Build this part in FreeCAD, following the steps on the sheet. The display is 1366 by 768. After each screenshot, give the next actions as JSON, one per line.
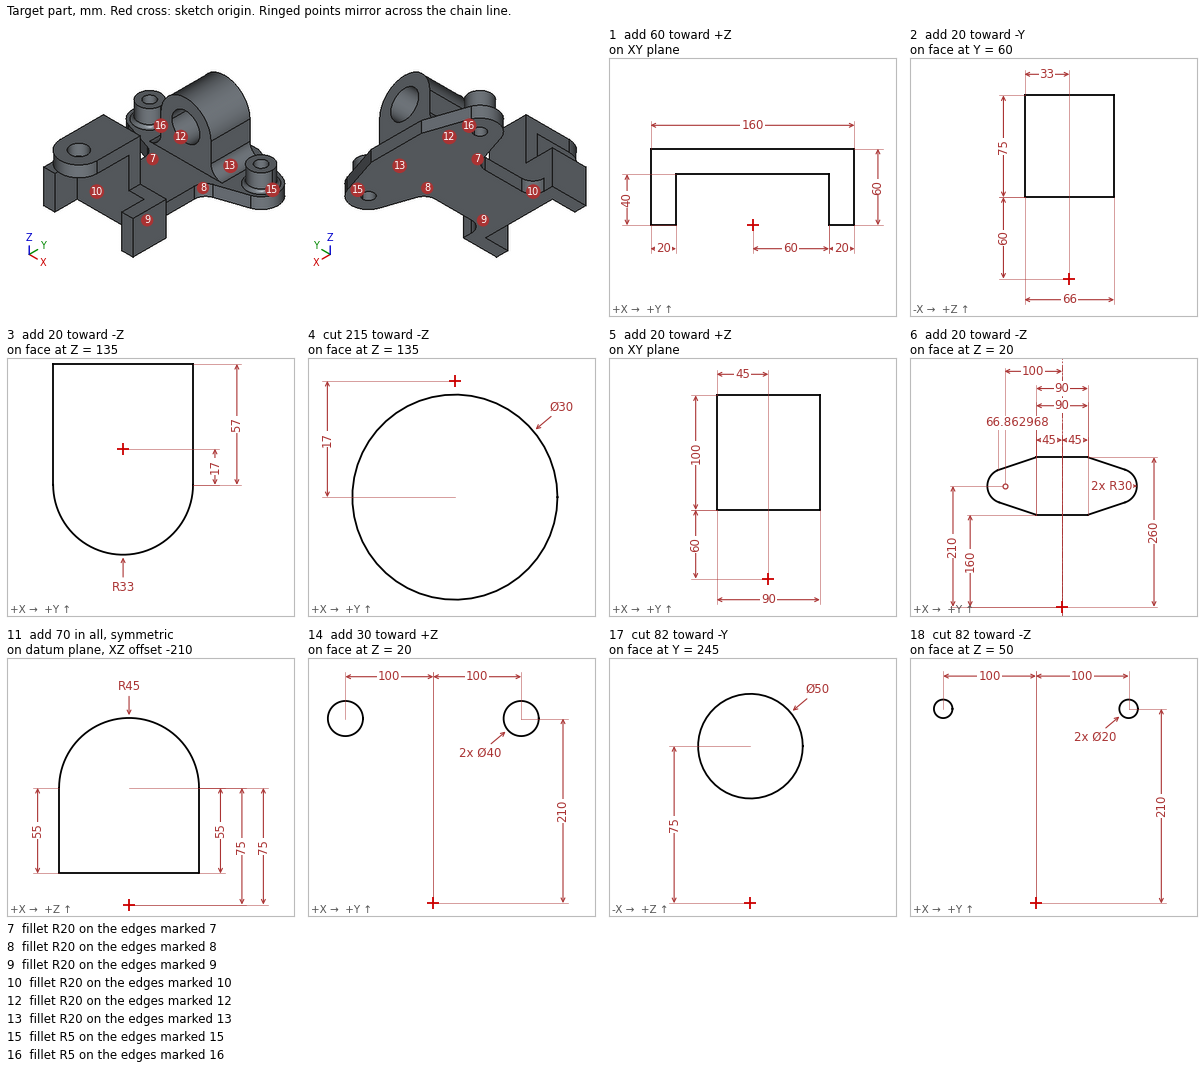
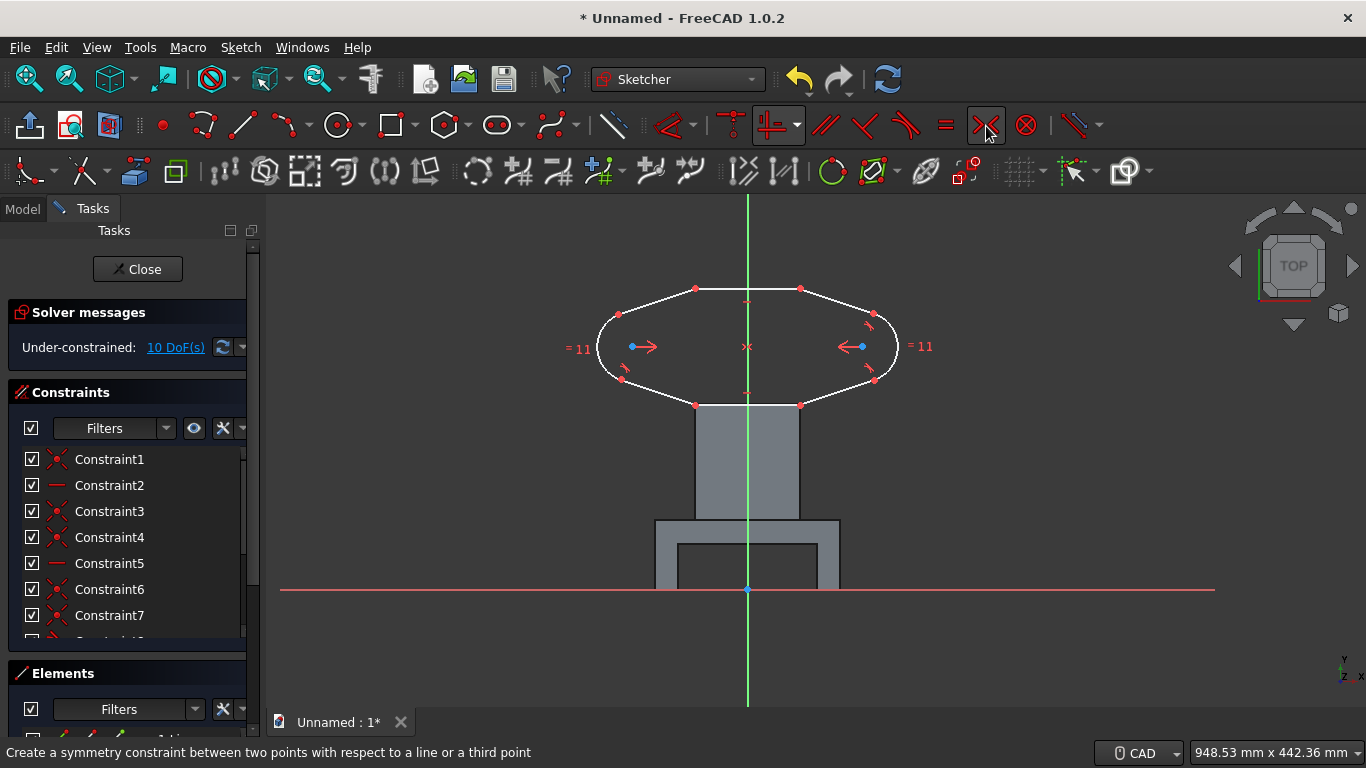
{"action": "key", "text": "d"}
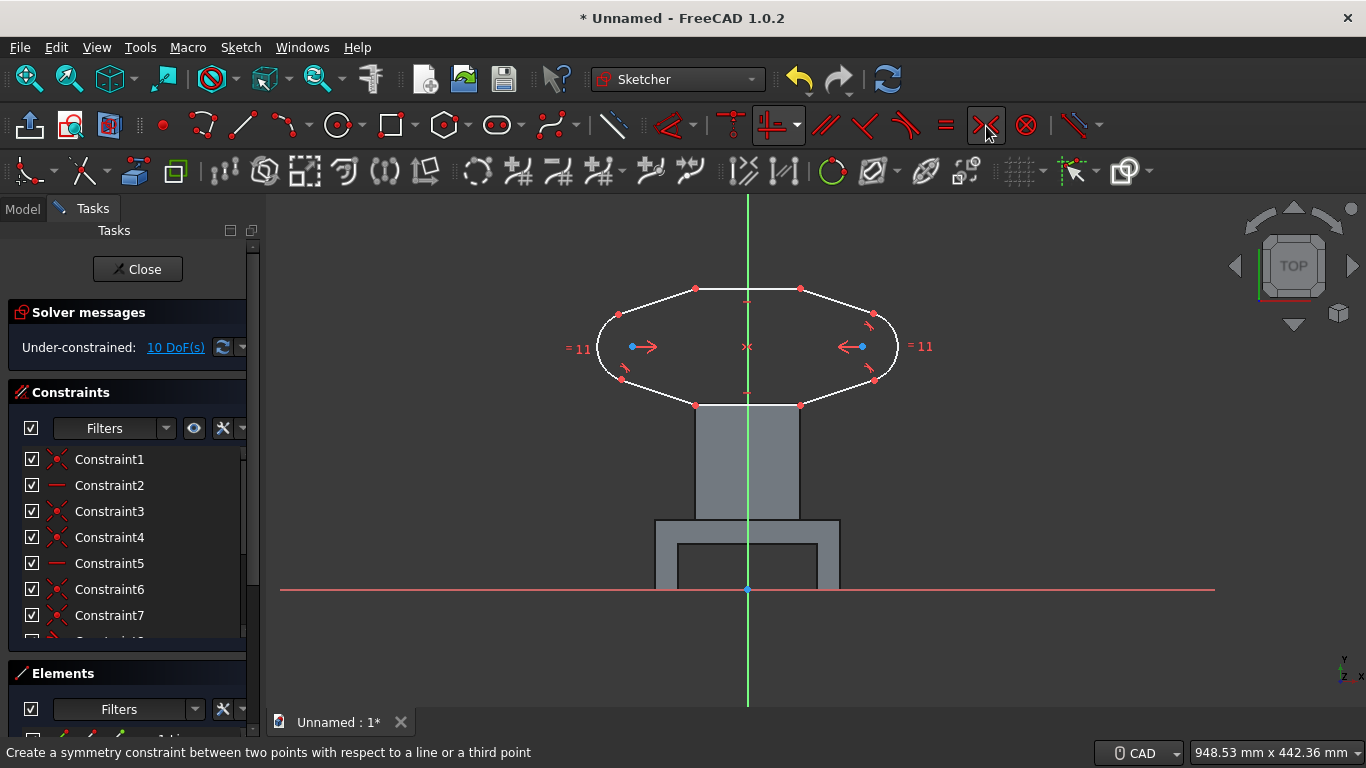
{"action": "left_click", "coordinate": [600, 332]}
{"action": "left_click", "coordinate": [571, 319]}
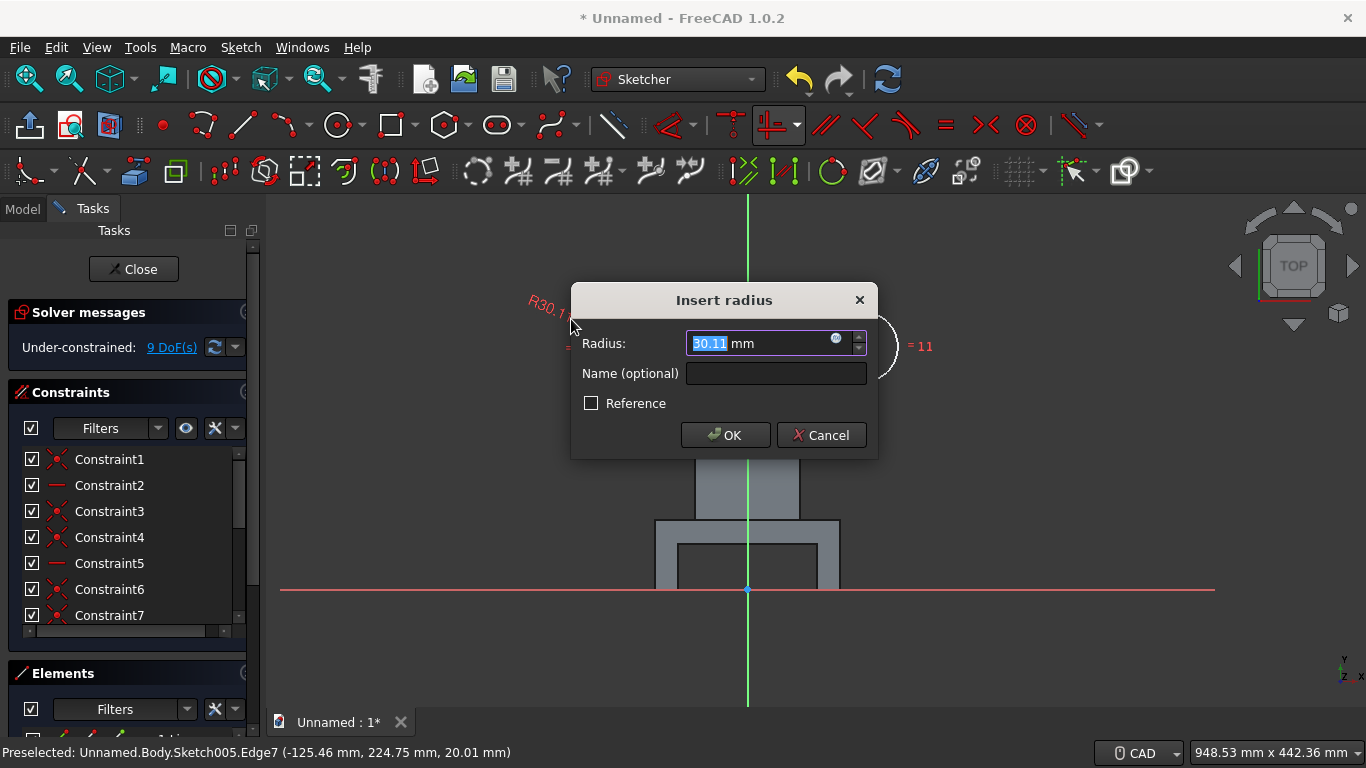
{"action": "type", "text": "30"}
{"action": "key", "text": "Return"}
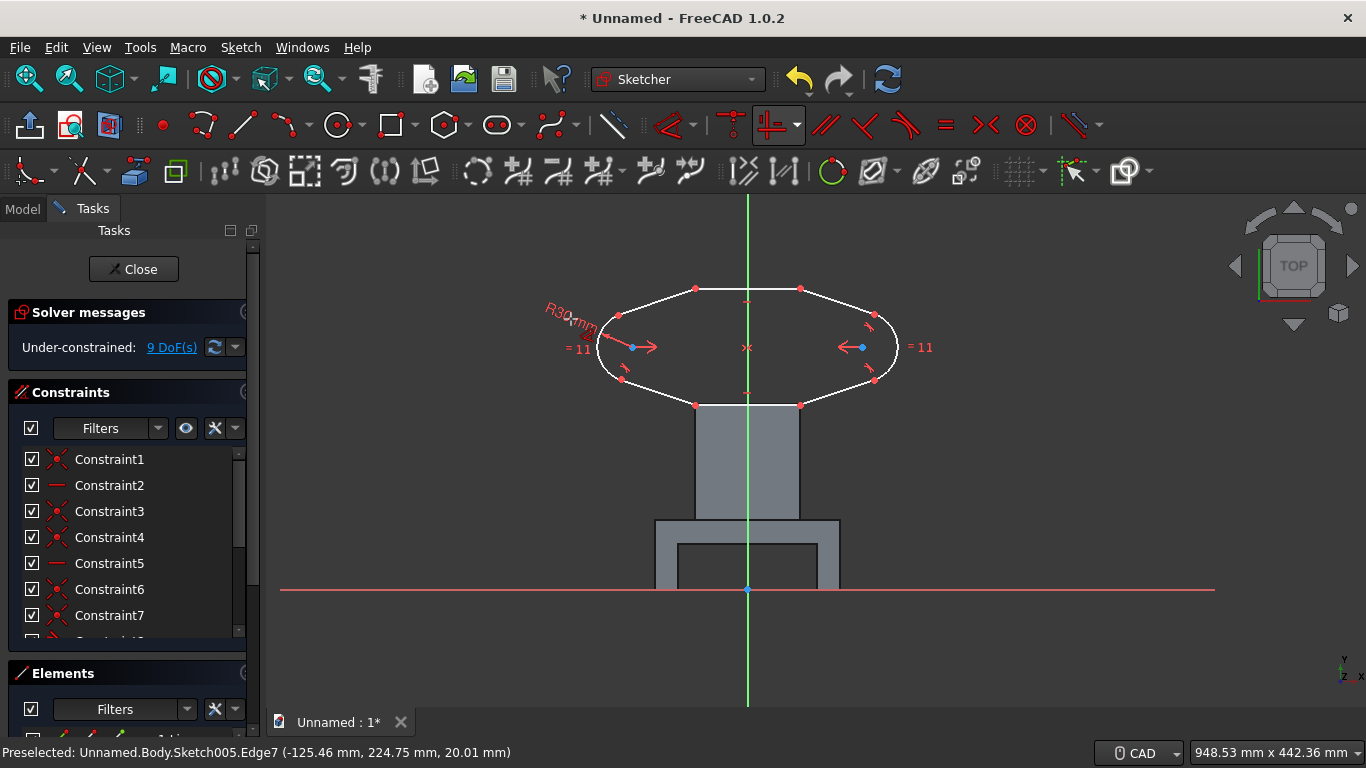
{"action": "left_click", "coordinate": [769, 289]}
{"action": "left_click", "coordinate": [723, 255]}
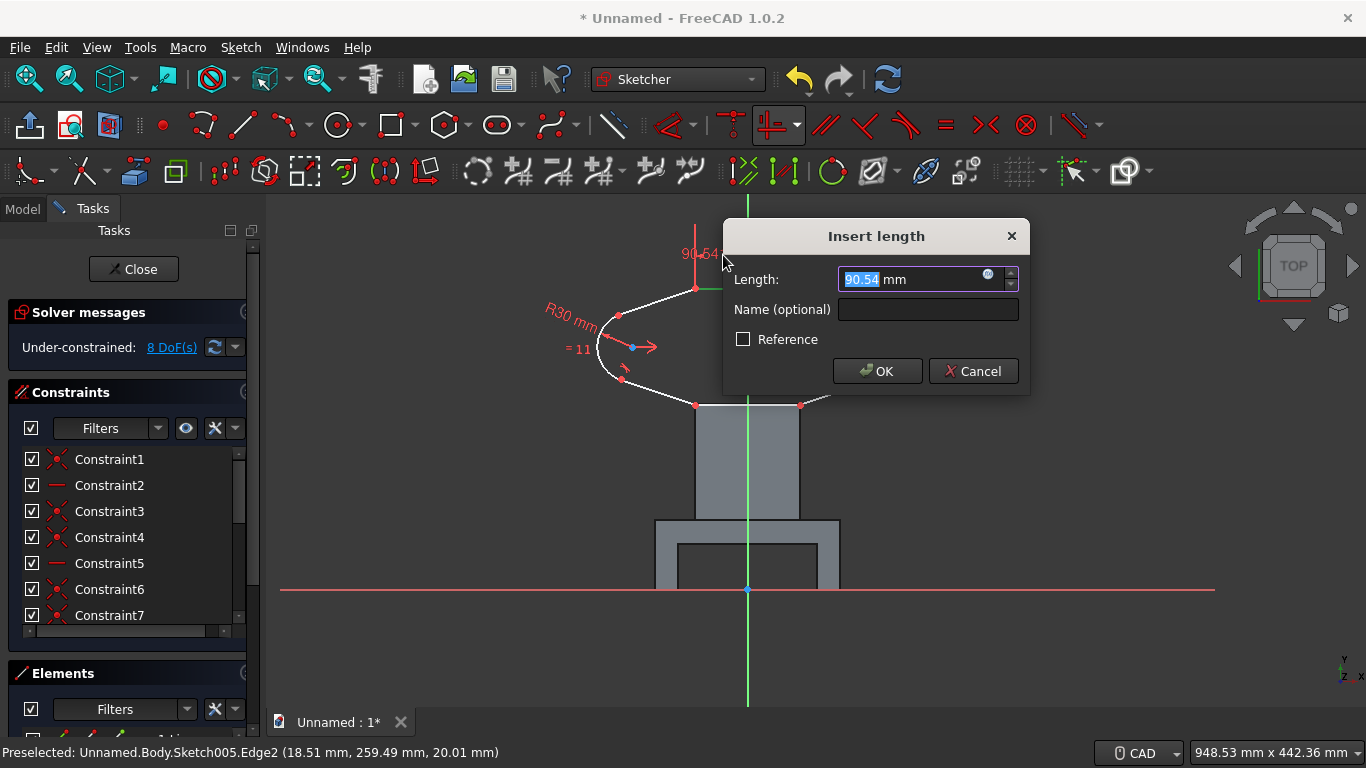
{"action": "type", "text": "90"}
{"action": "key", "text": "Return"}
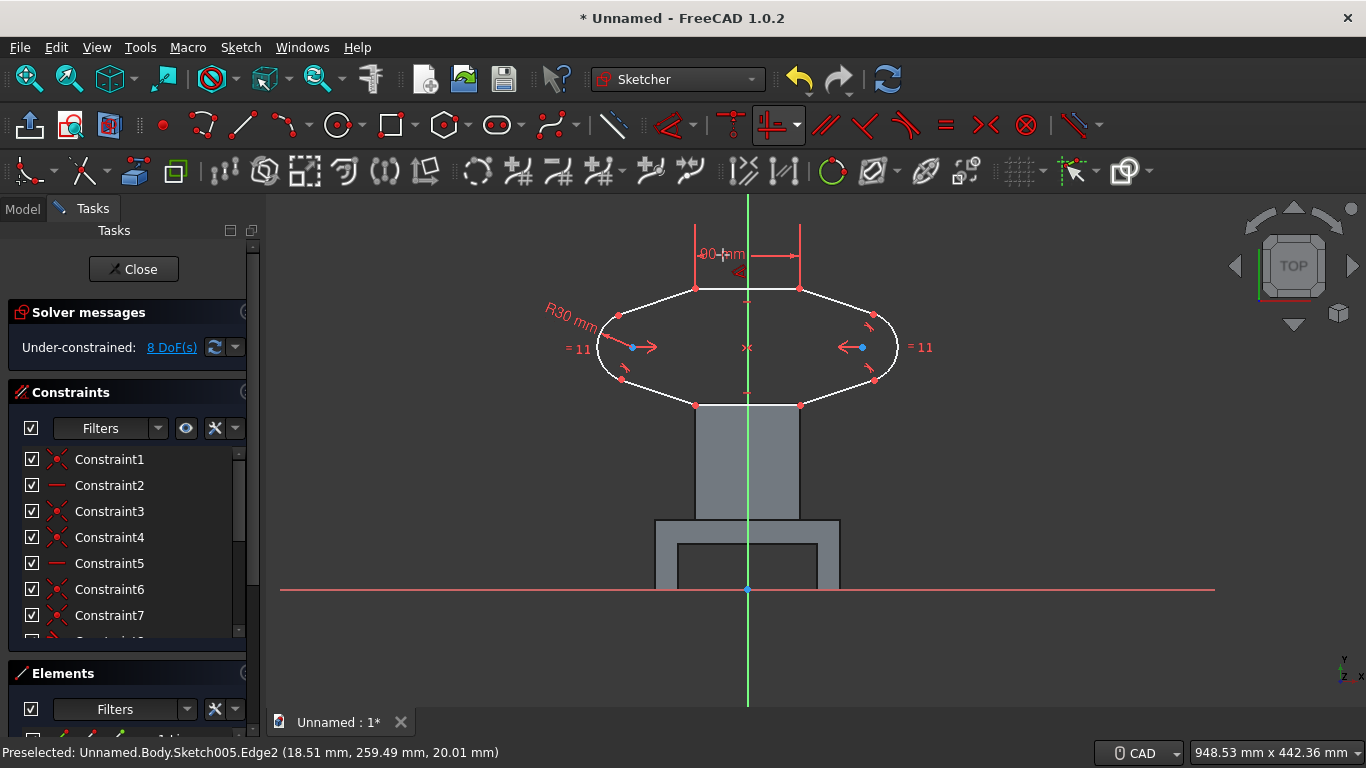
{"action": "left_click", "coordinate": [727, 405]}
{"action": "left_click", "coordinate": [723, 371]}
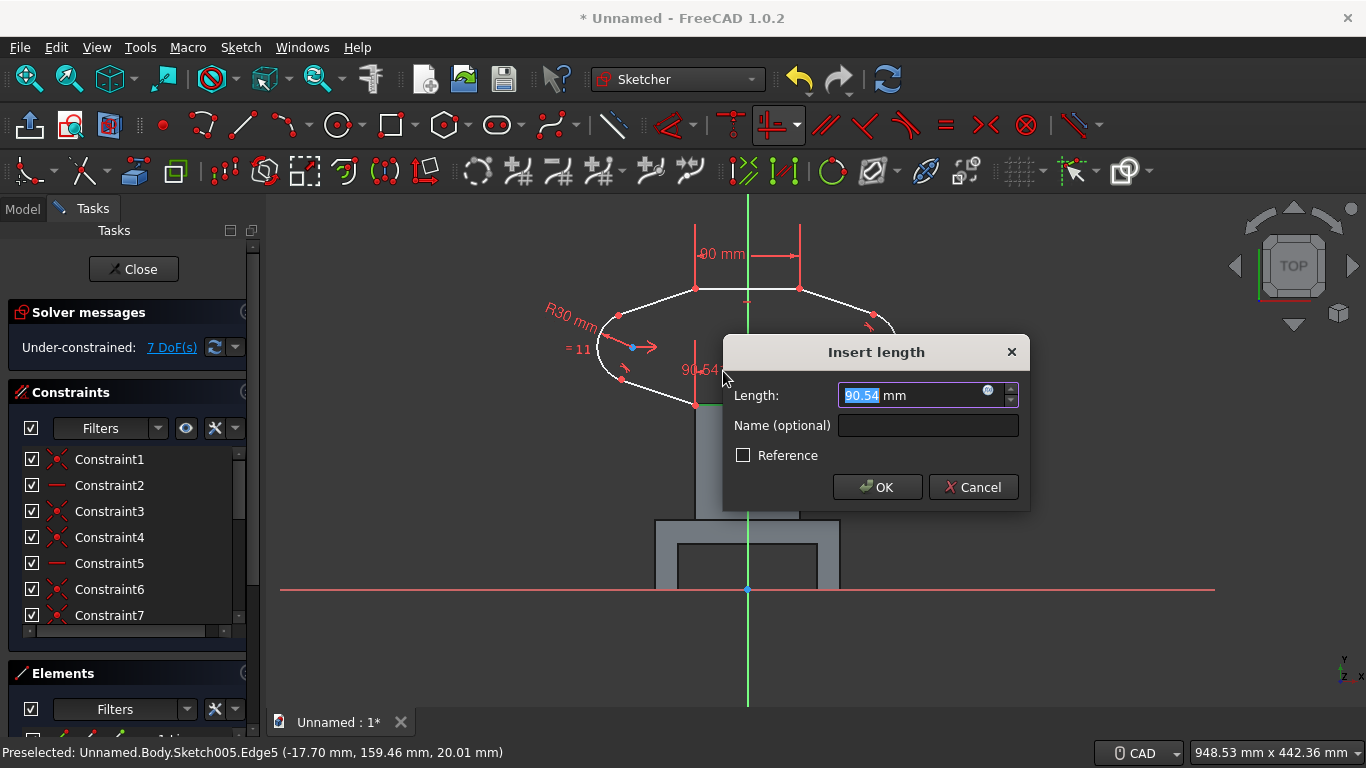
{"action": "type", "text": "90"}
{"action": "key", "text": "Return"}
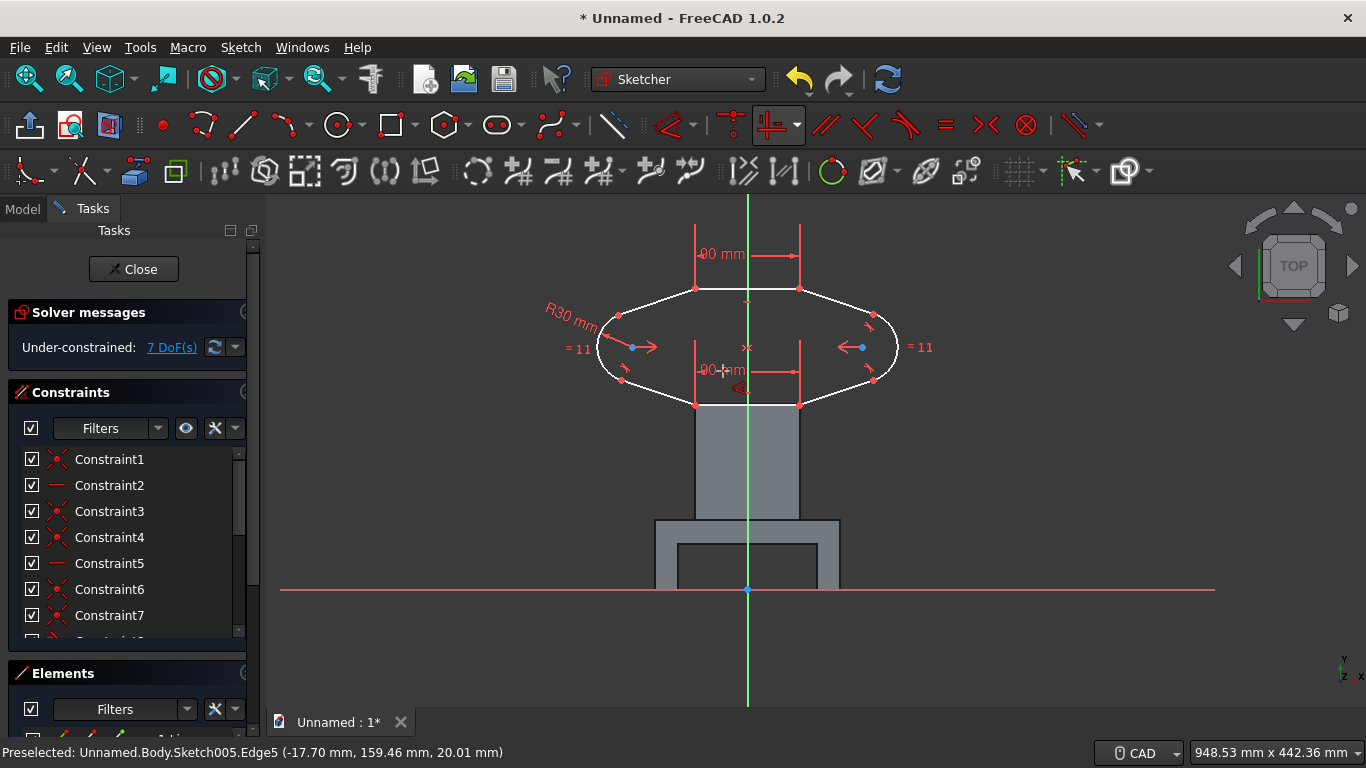
{"action": "left_click", "coordinate": [800, 289]}
{"action": "left_click", "coordinate": [774, 624]}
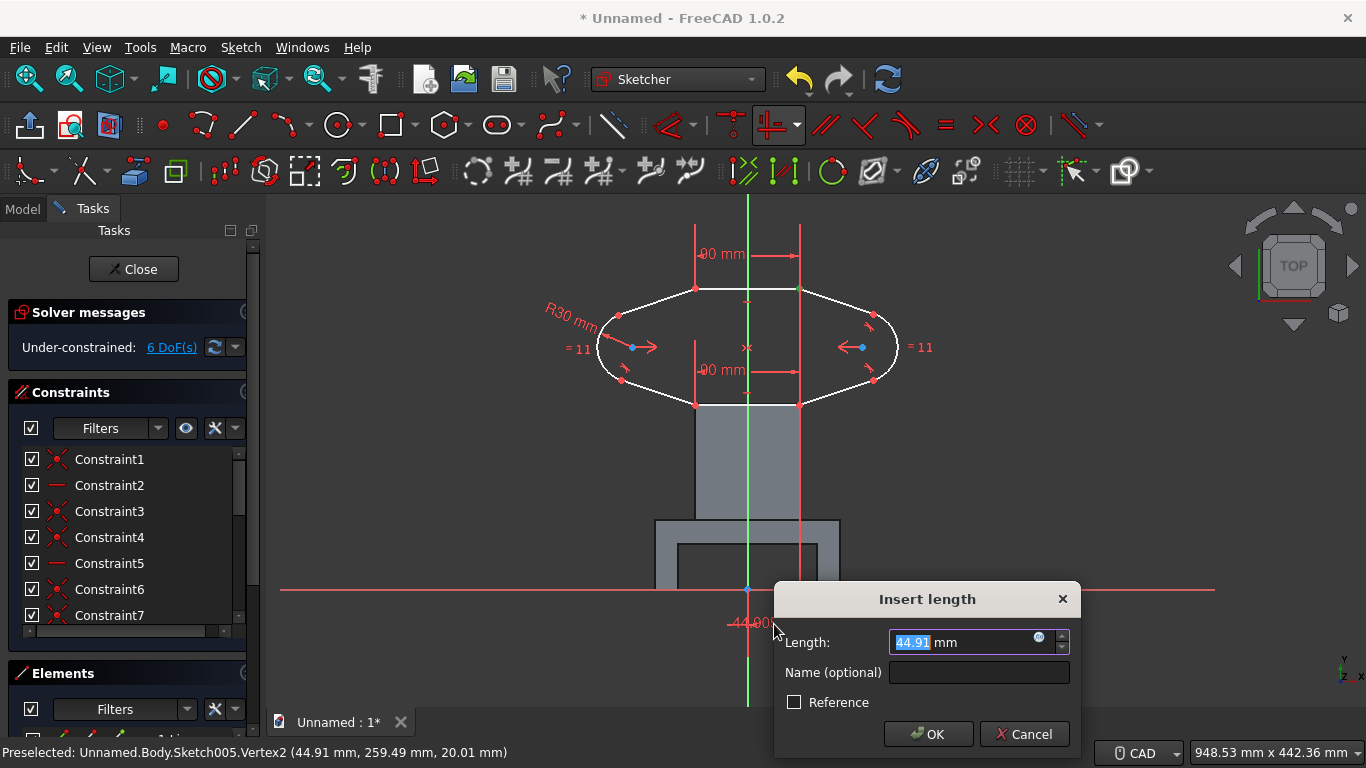
{"action": "type", "text": "45"}
{"action": "key", "text": "Return"}